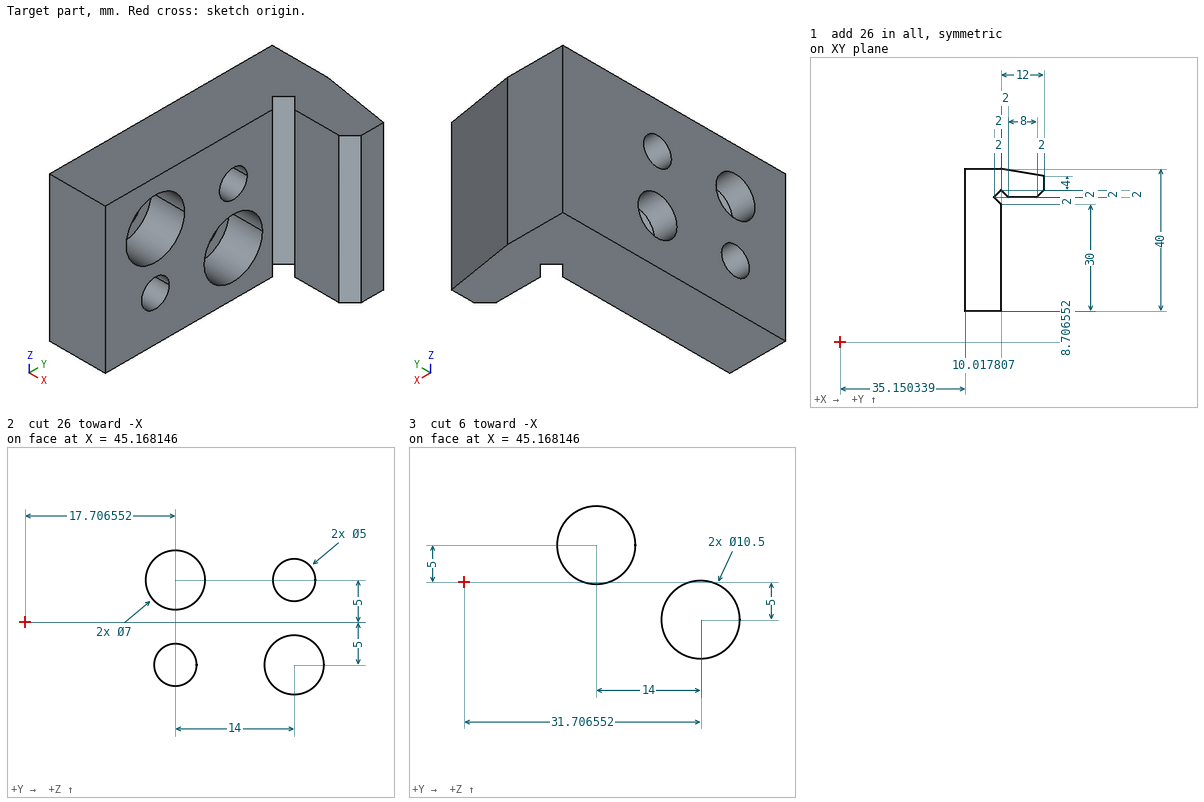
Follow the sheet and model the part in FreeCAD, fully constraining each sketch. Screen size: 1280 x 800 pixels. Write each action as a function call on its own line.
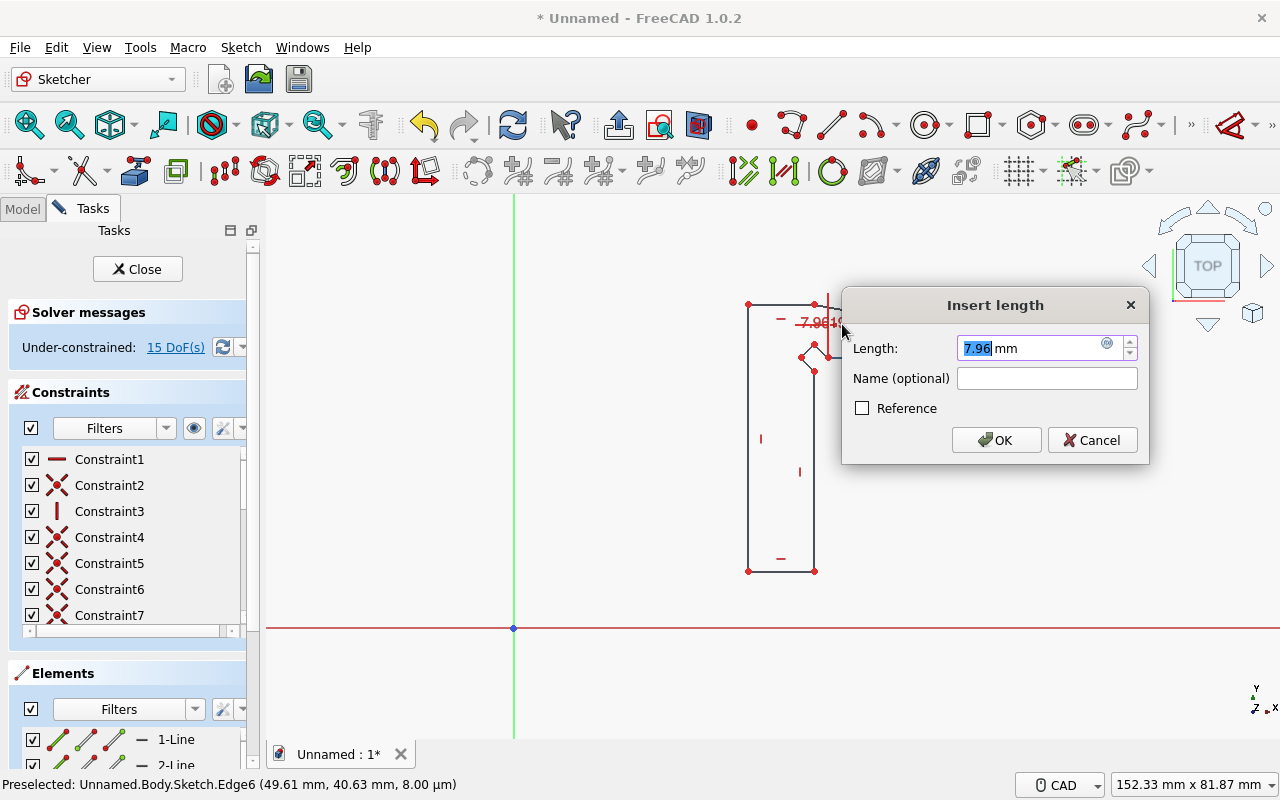
text(8)
key(Return)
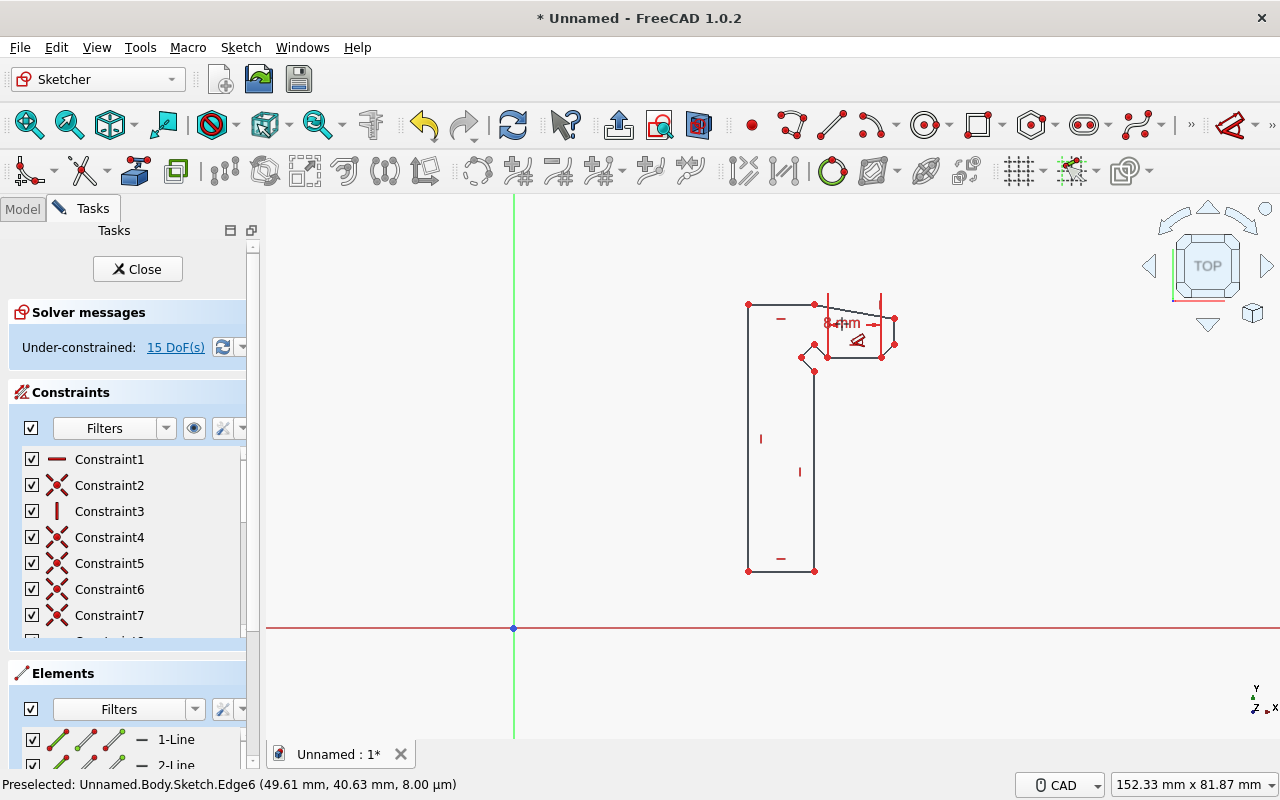
scroll(894, 335, up, 2)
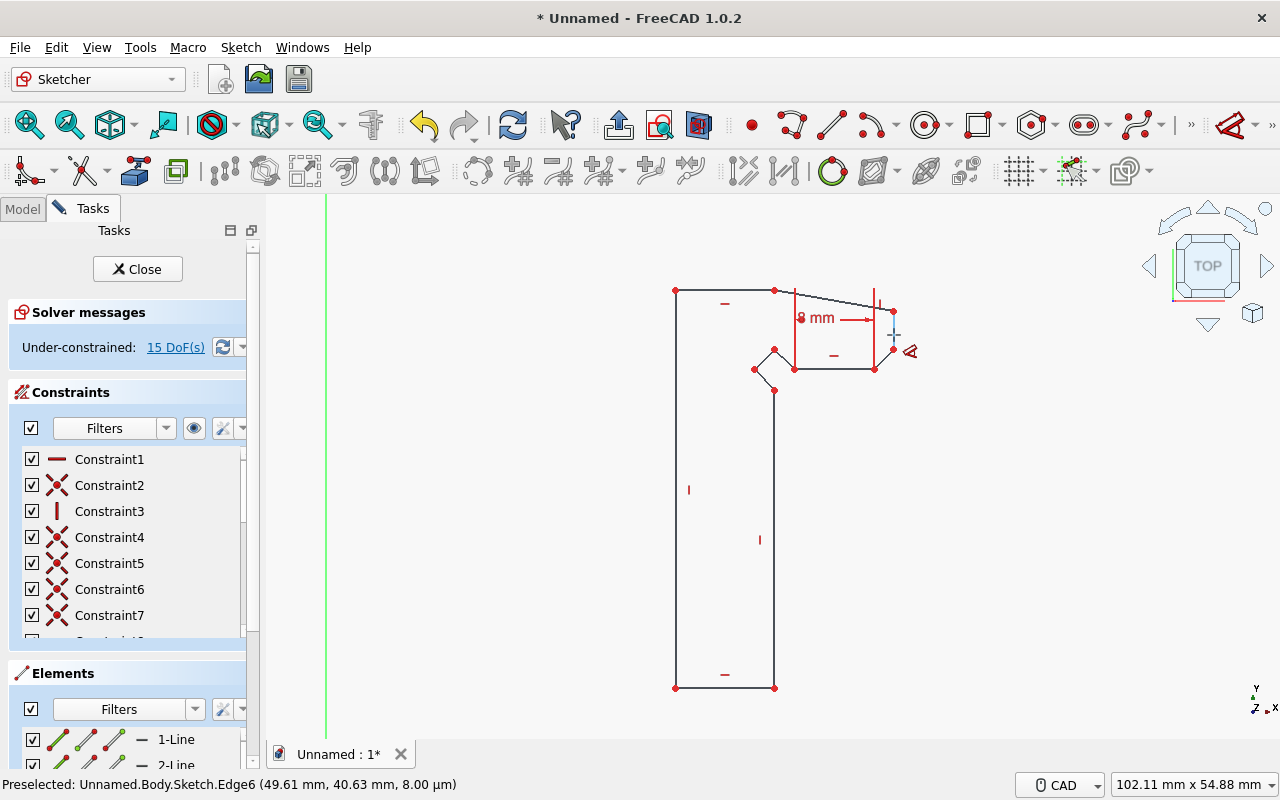
click(894, 334)
click(928, 330)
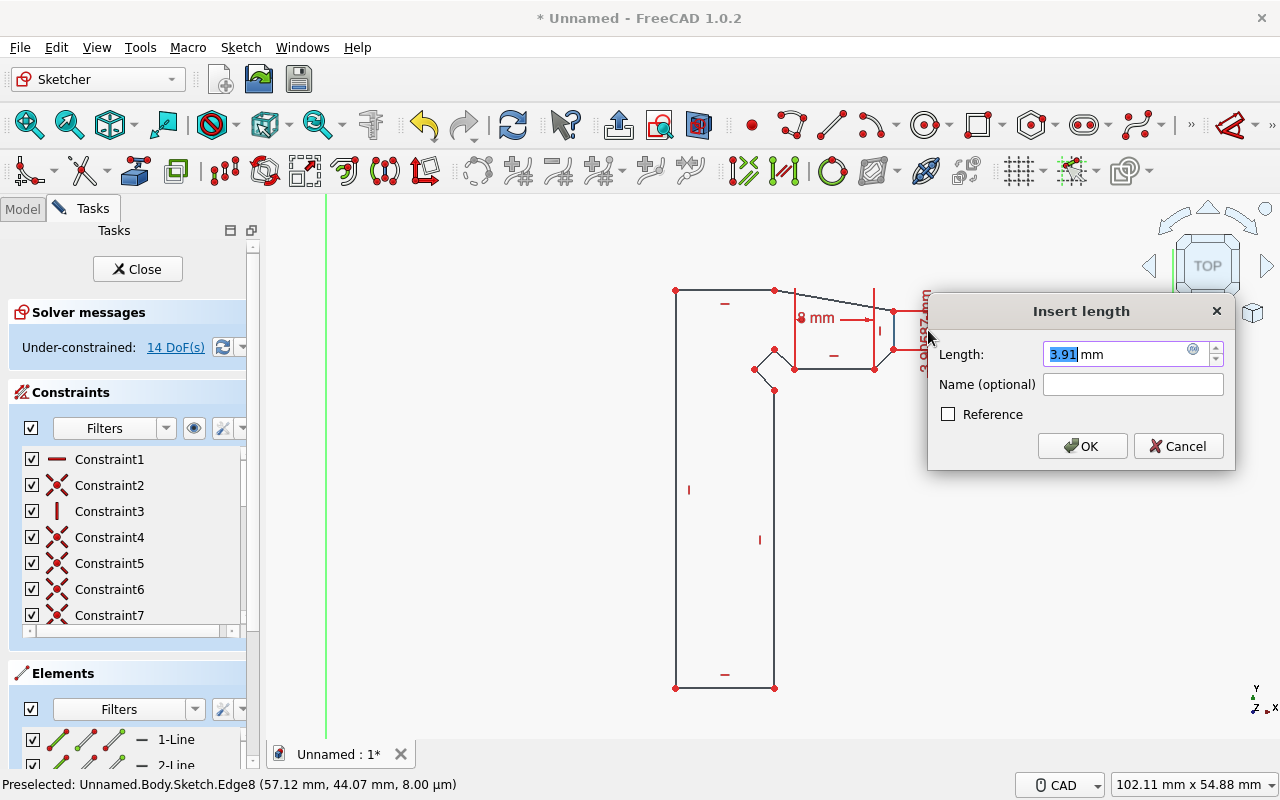
text(4)
key(Return)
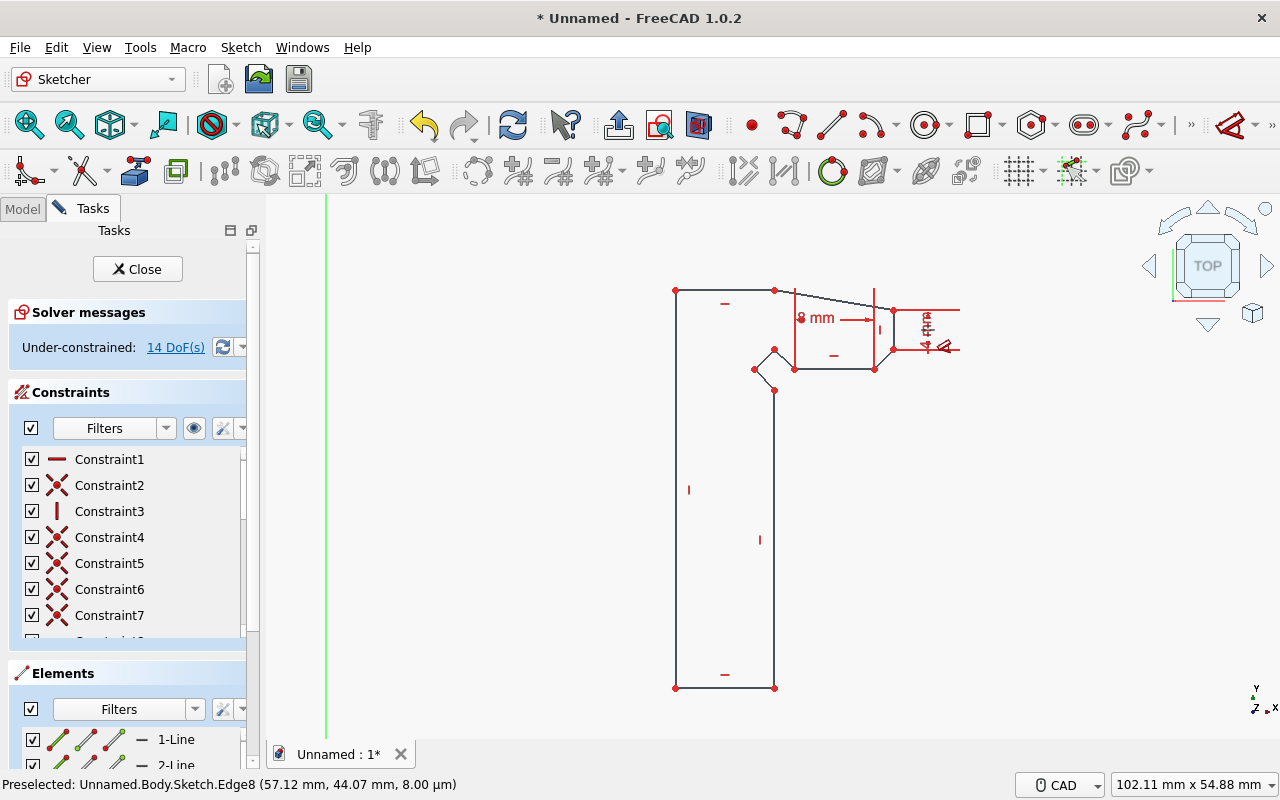
click(774, 599)
click(808, 539)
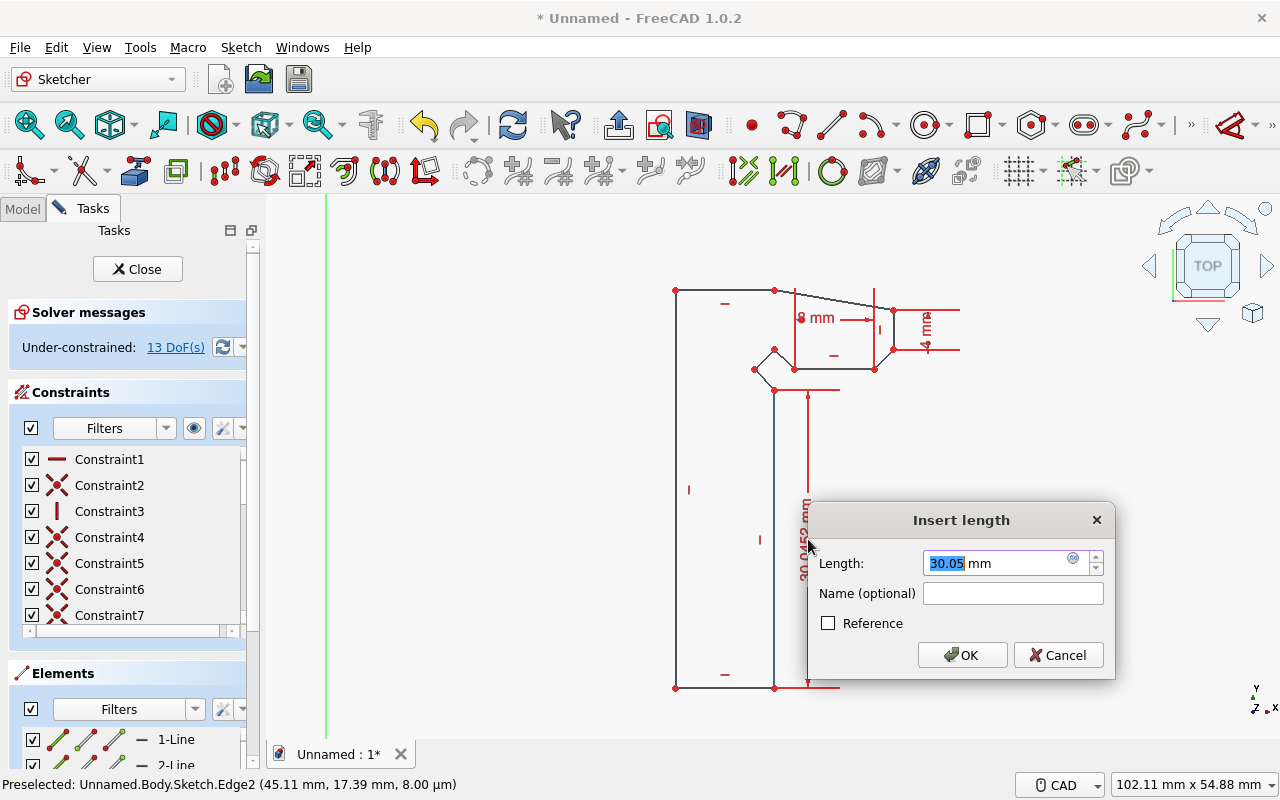
text(30)
key(Return)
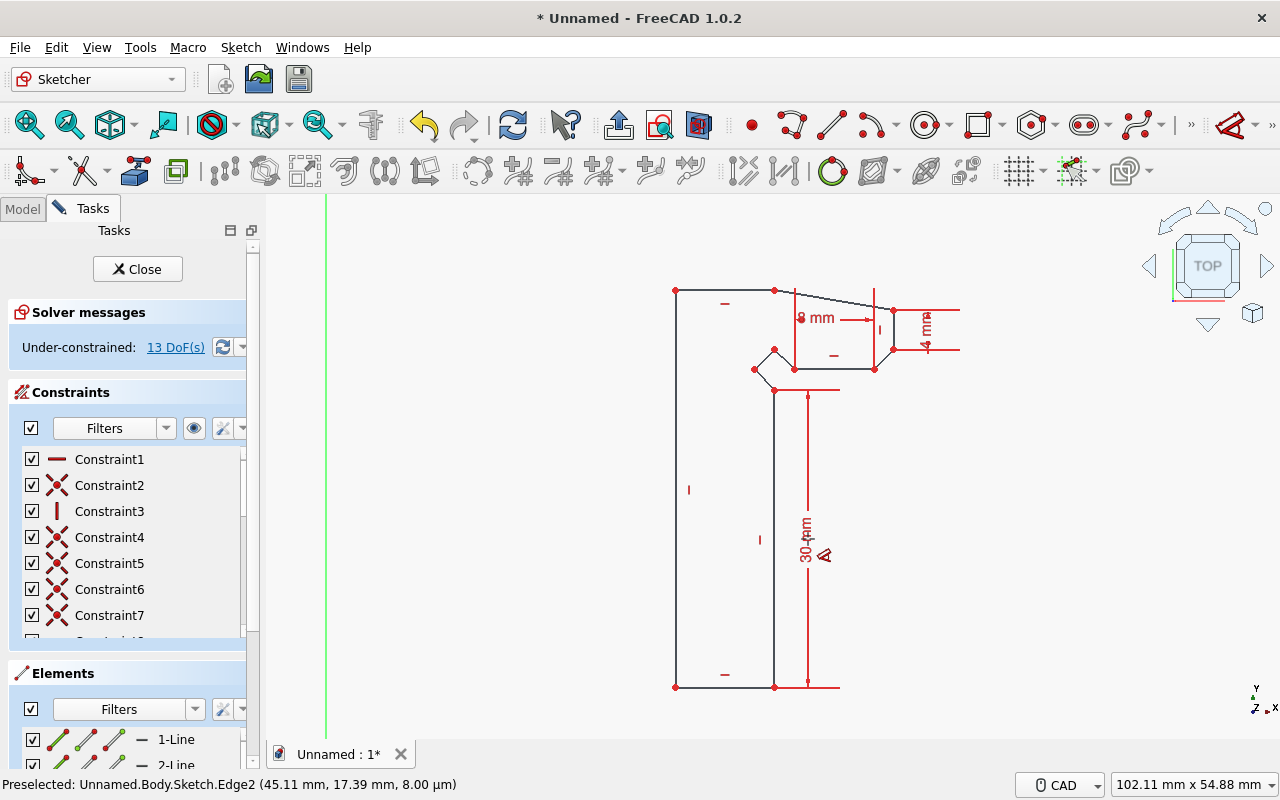
click(676, 409)
click(710, 489)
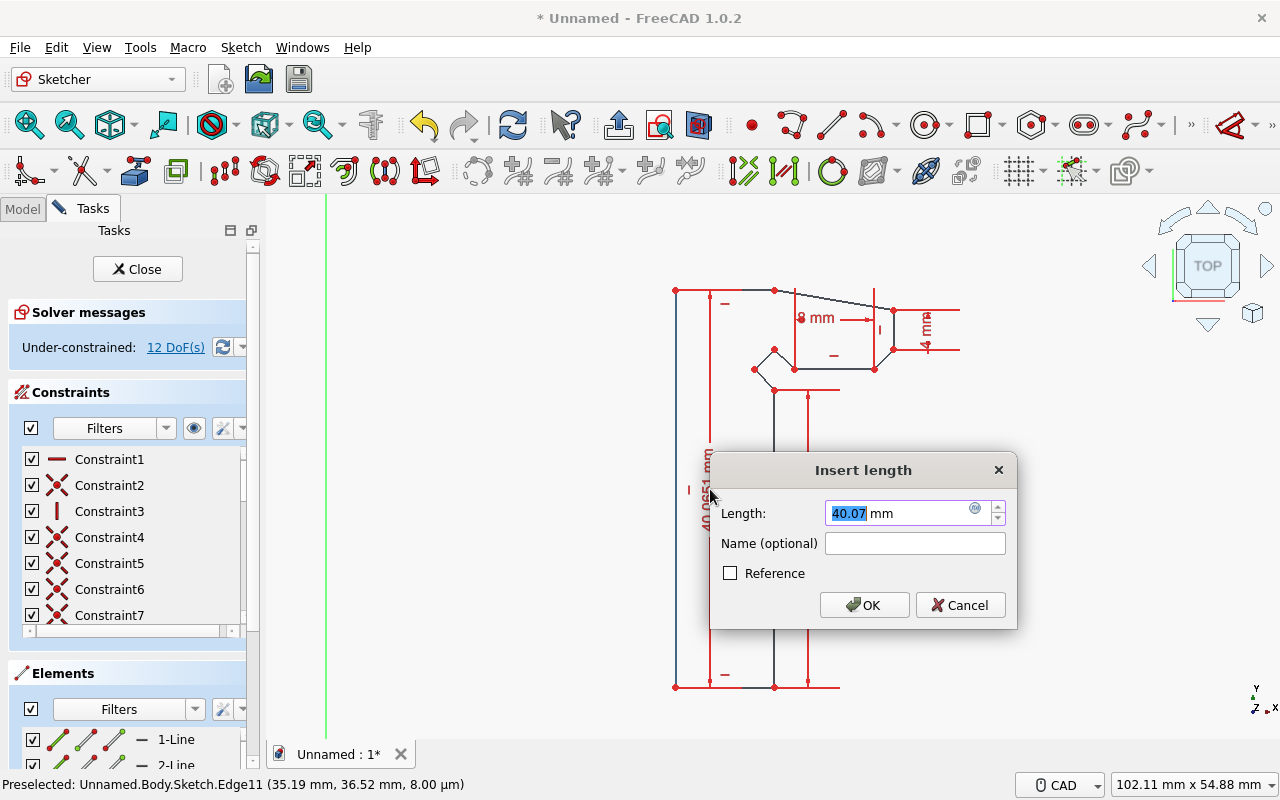
text(40)
key(Return)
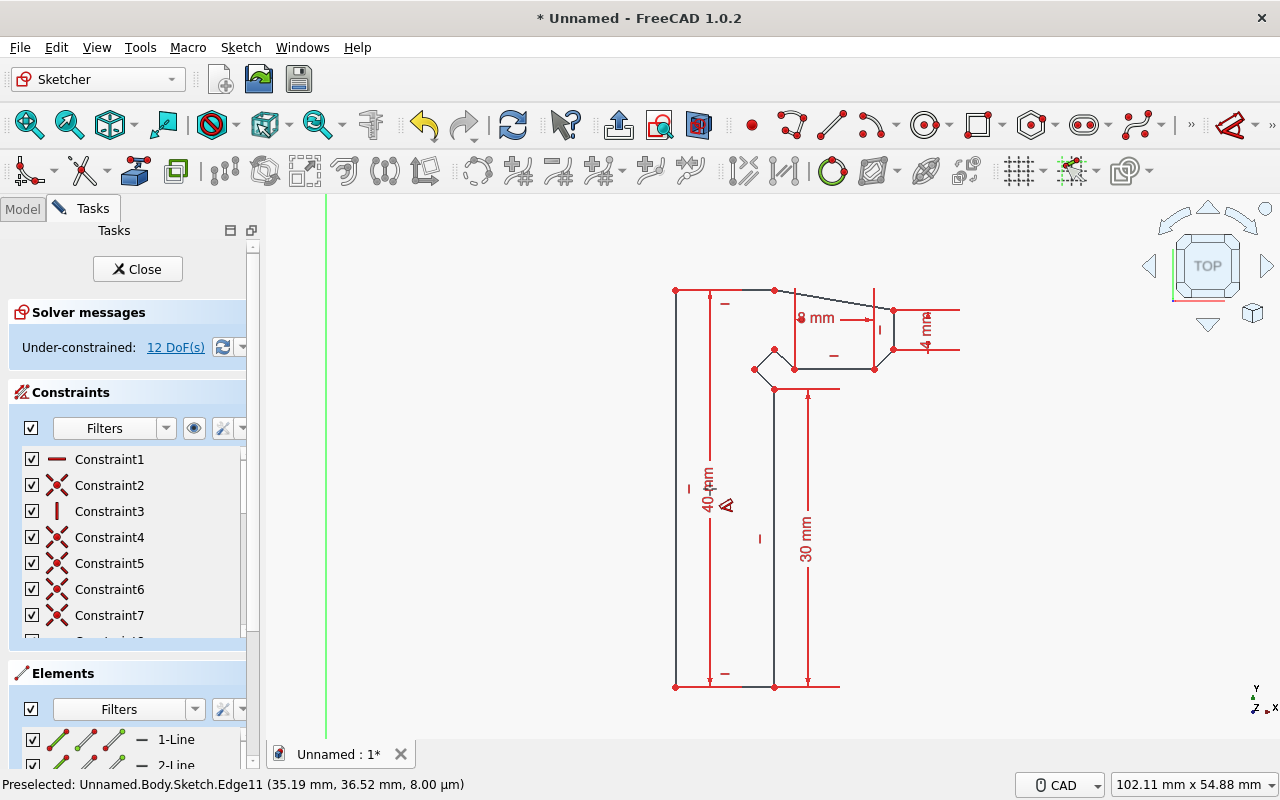
scroll(767, 381, up, 4)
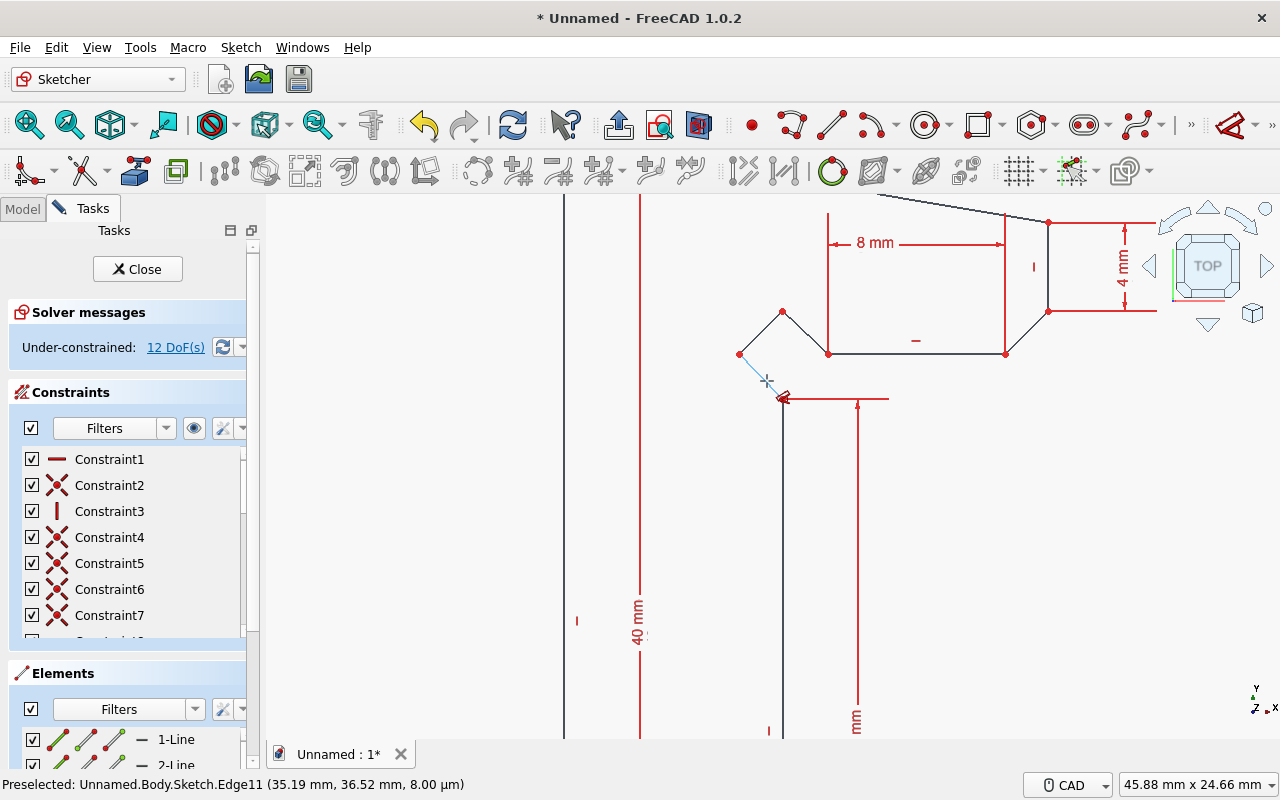
click(765, 381)
click(751, 320)